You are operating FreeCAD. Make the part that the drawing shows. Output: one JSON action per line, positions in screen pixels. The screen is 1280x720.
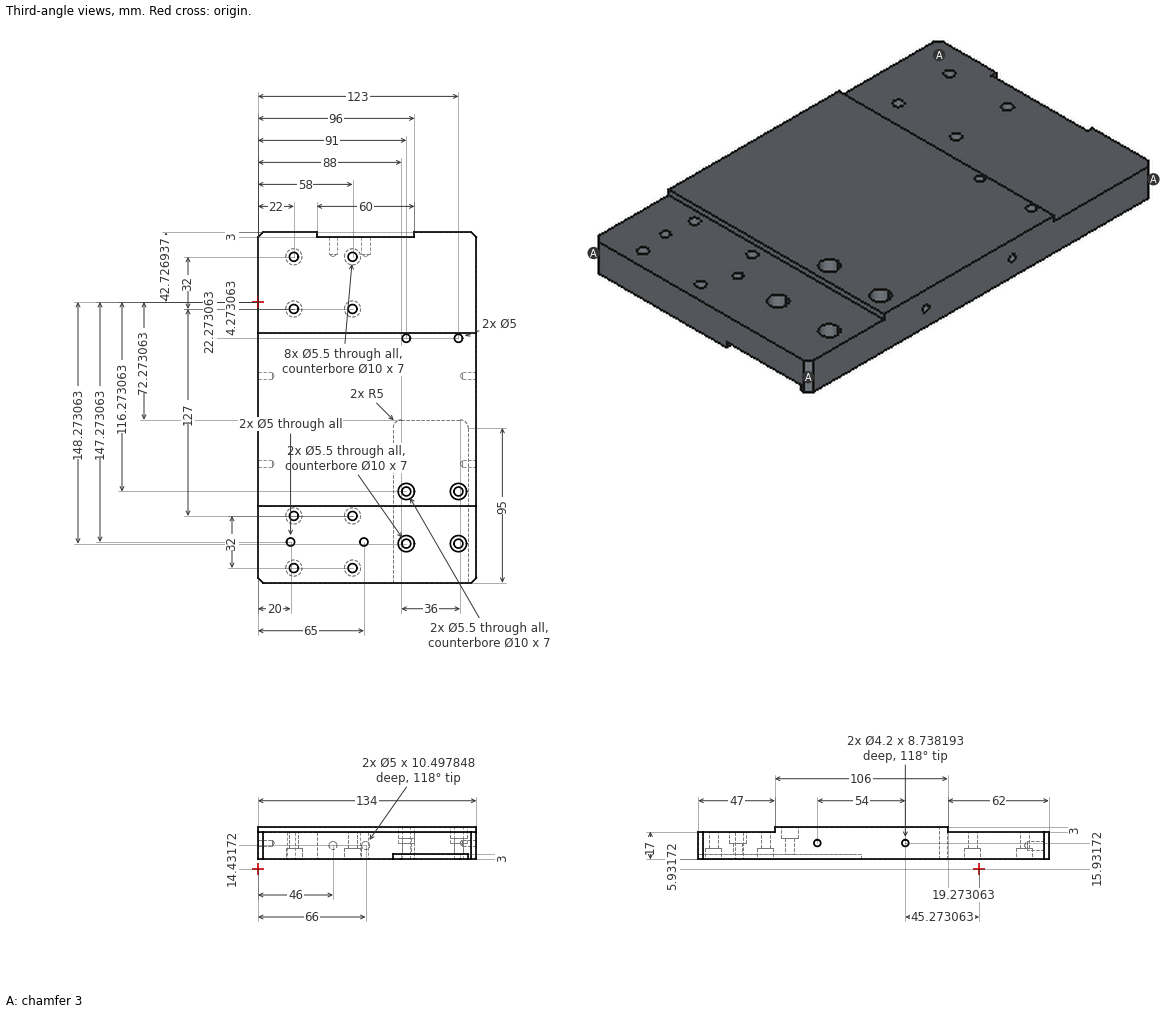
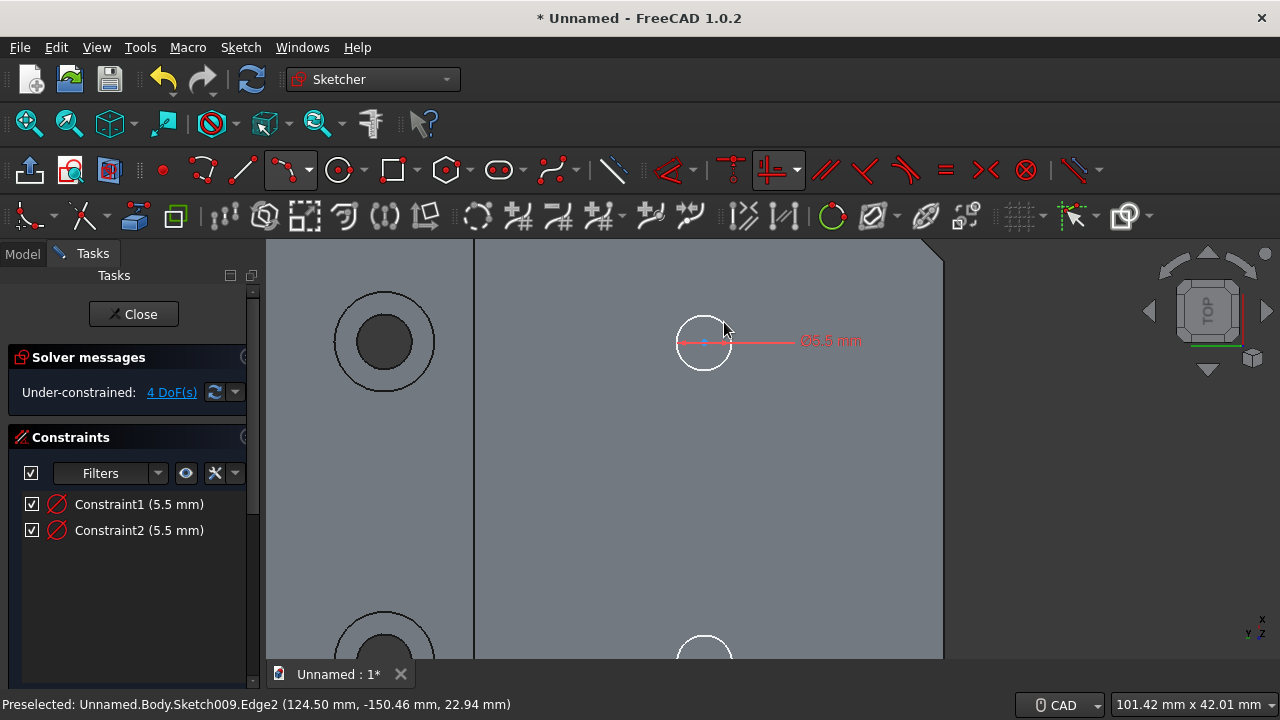
{"action": "scroll", "coordinate": [705, 342], "scroll_direction": "down", "scroll_amount": 2}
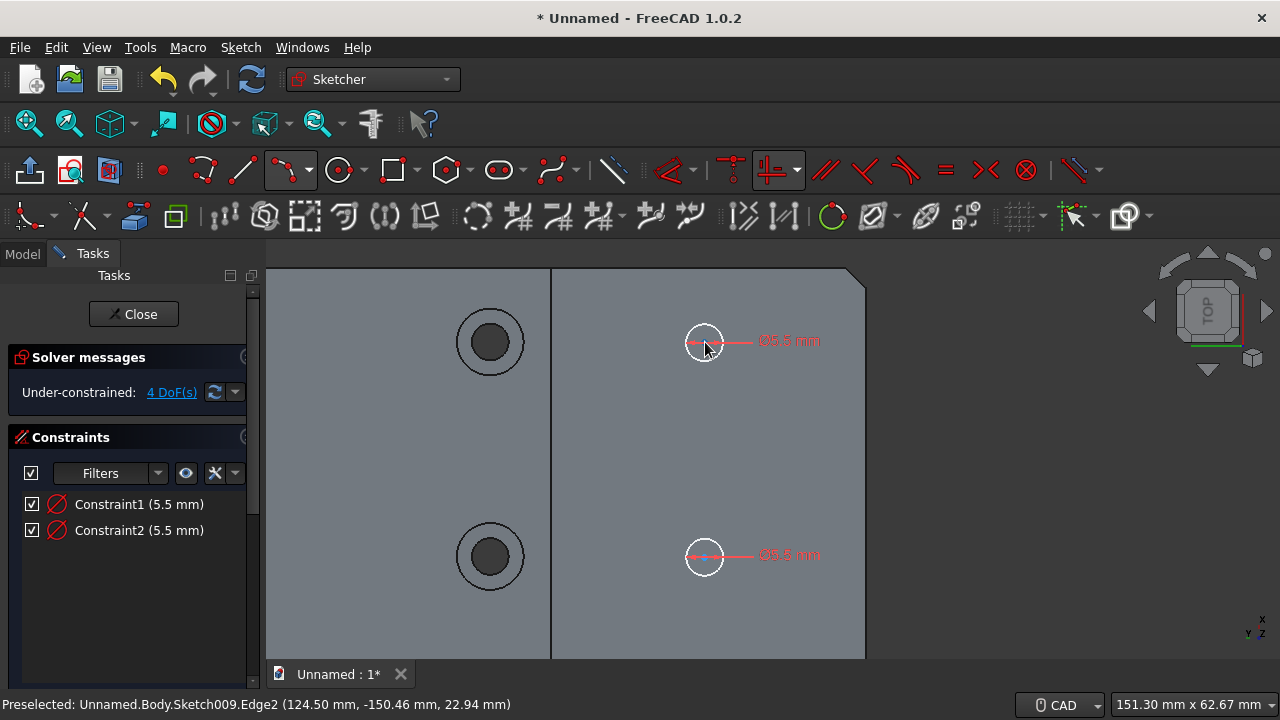
{"action": "left_click", "coordinate": [705, 557]}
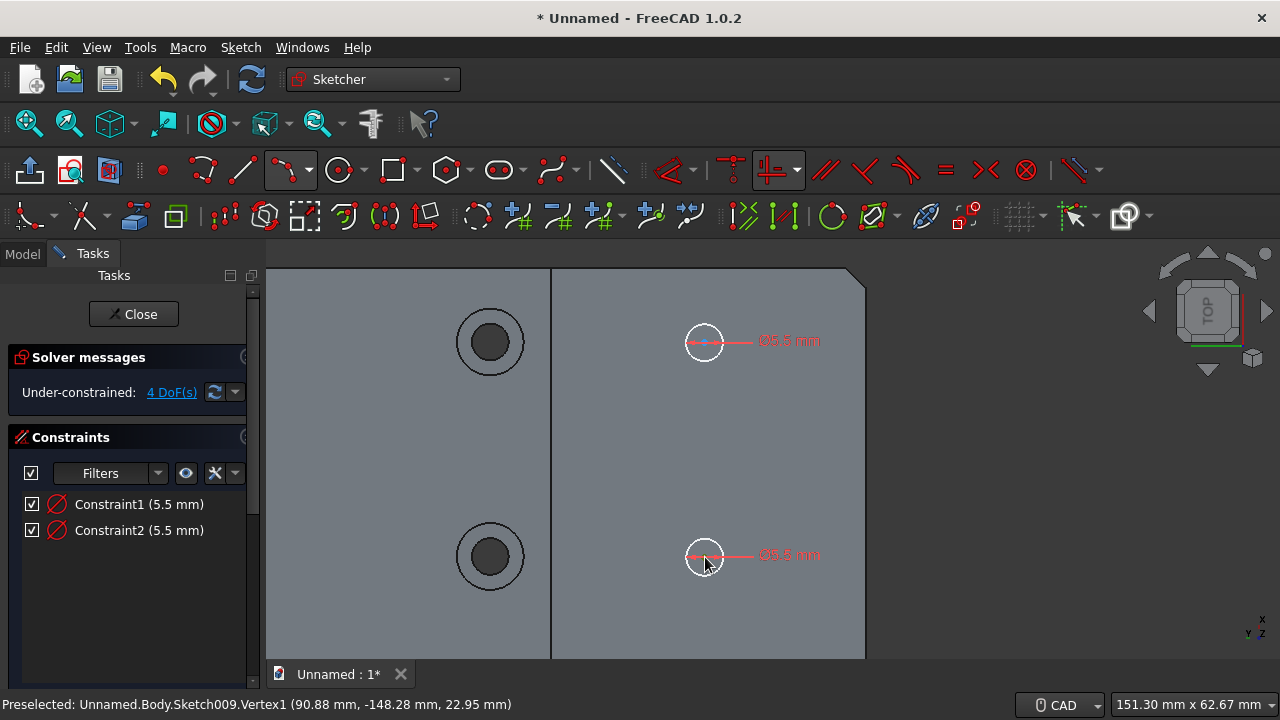
{"action": "left_click", "coordinate": [704, 343]}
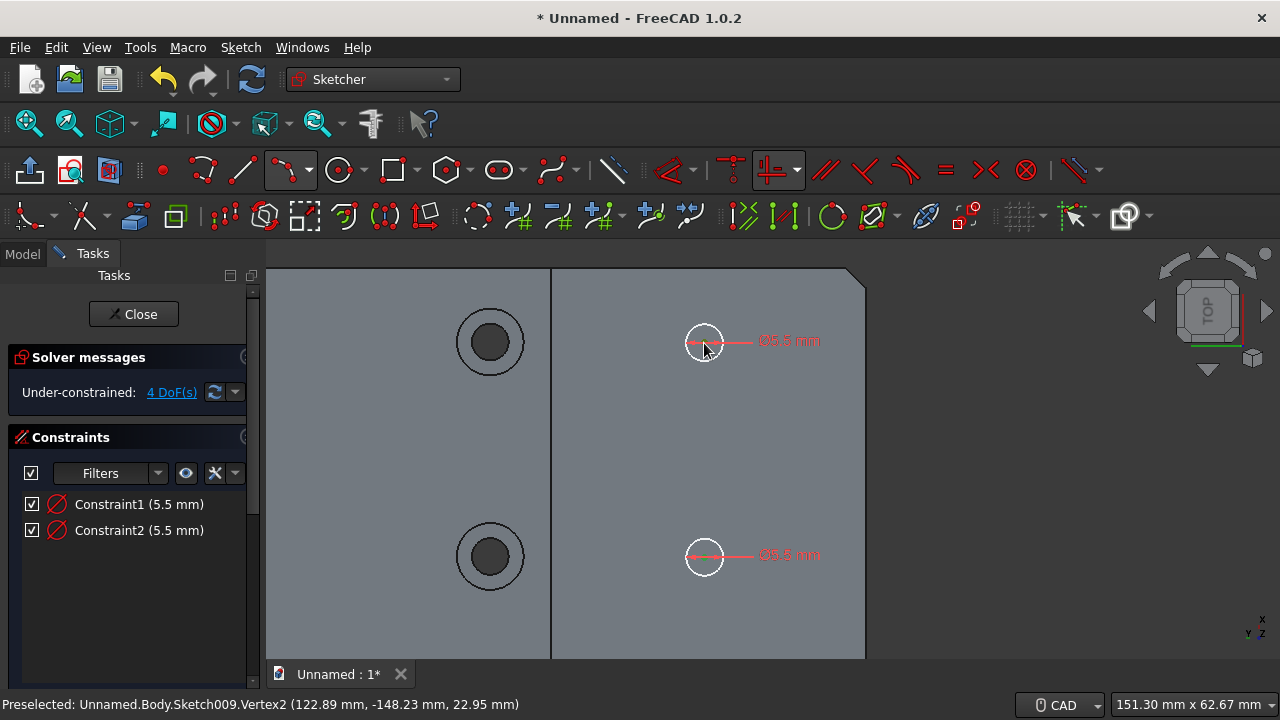
{"action": "key", "text": "v"}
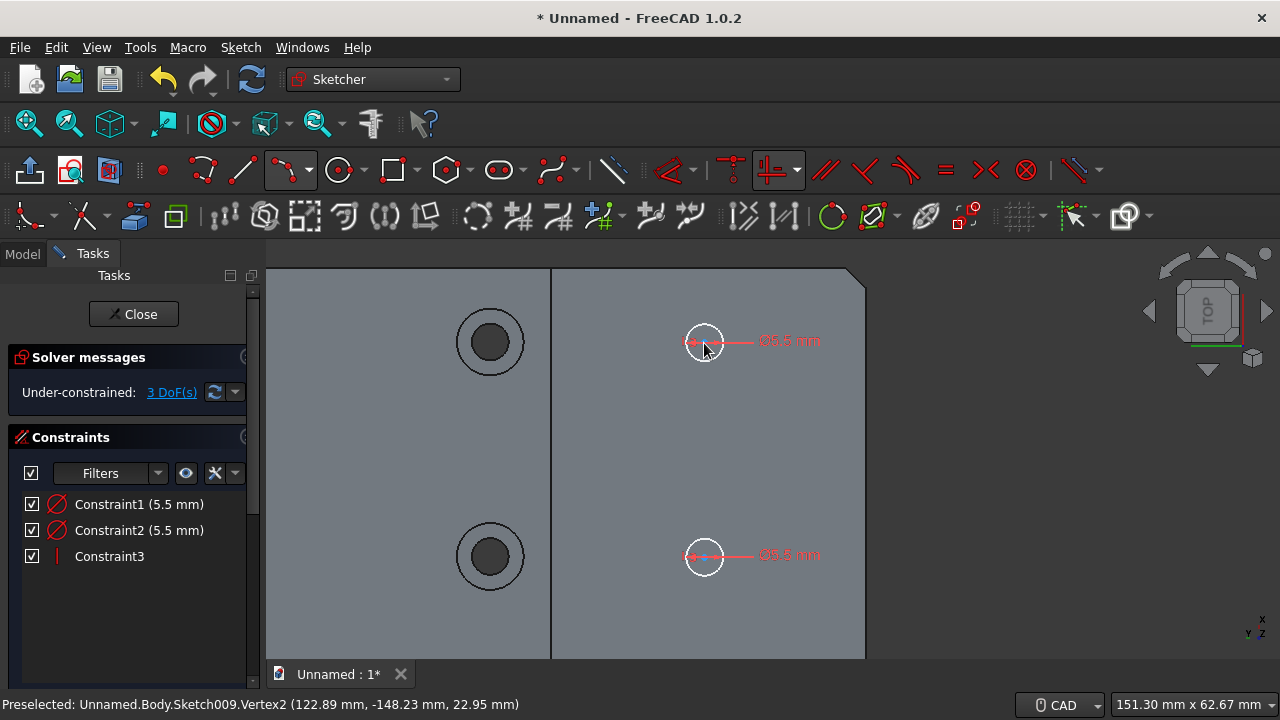
{"action": "left_click", "coordinate": [668, 170]}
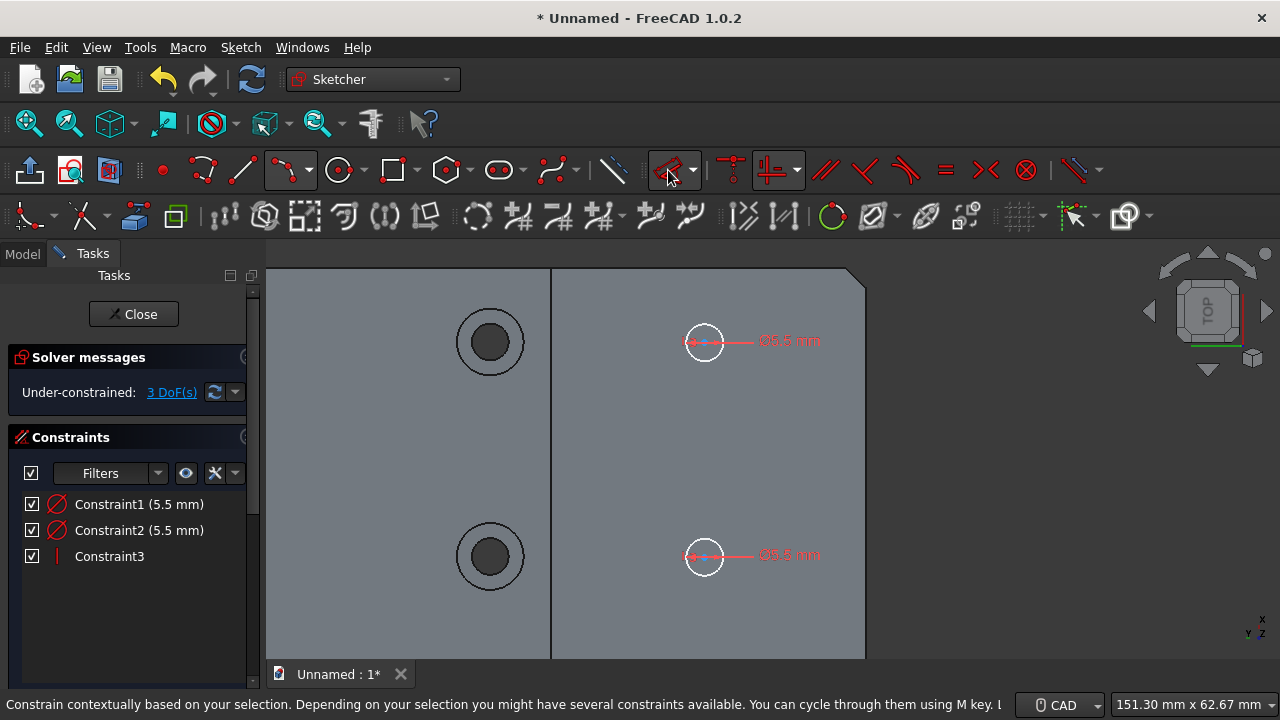
{"action": "left_click", "coordinate": [705, 557]}
{"action": "left_click", "coordinate": [739, 594]}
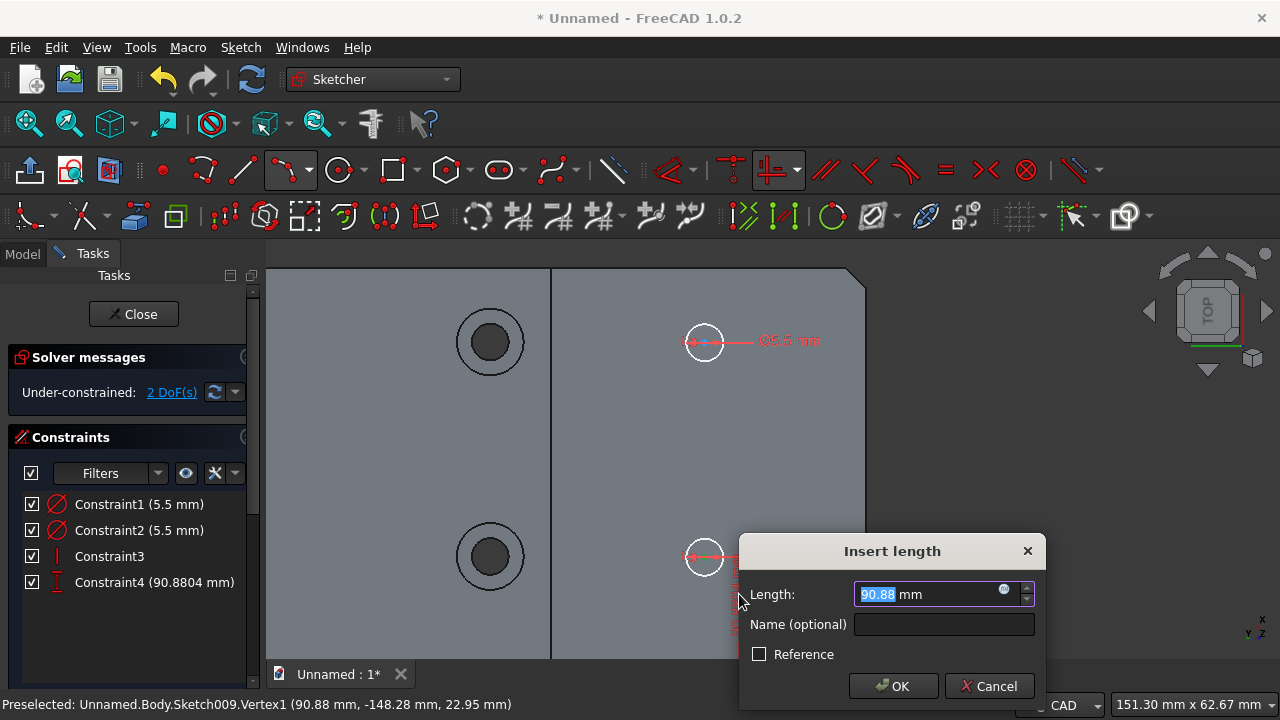
{"action": "type", "text": "91"}
{"action": "key", "text": "Return"}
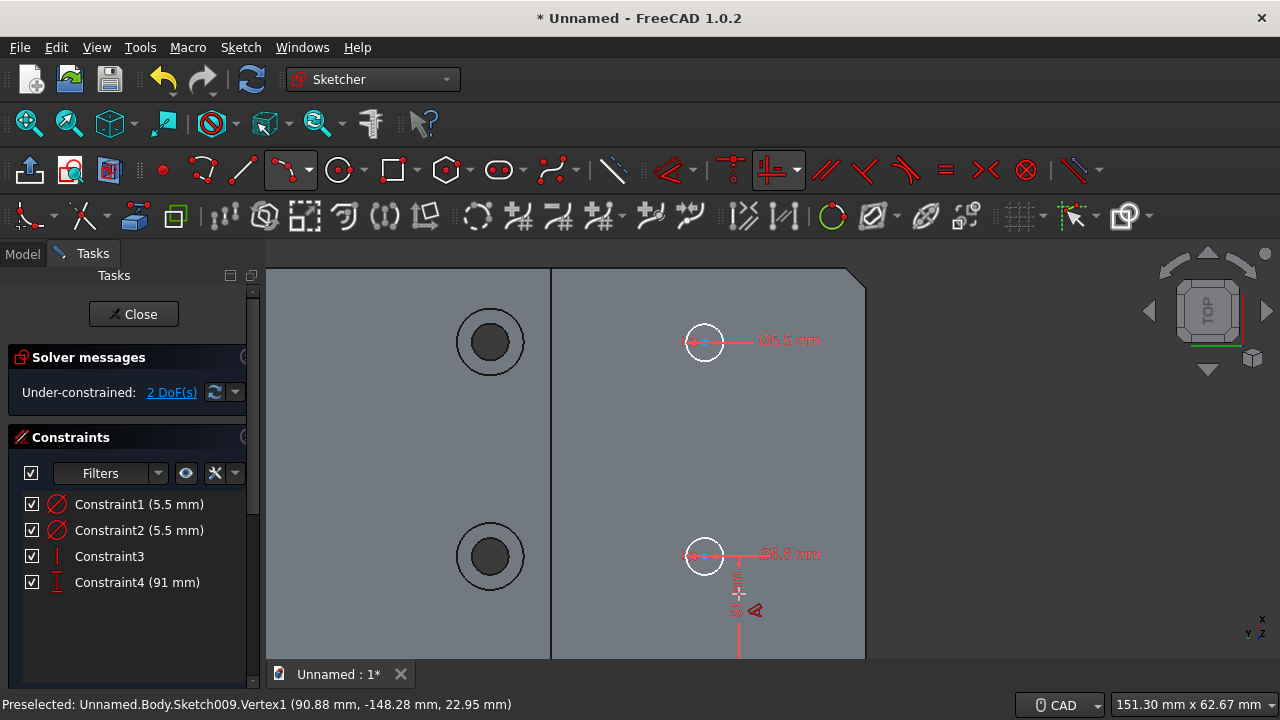
{"action": "left_click", "coordinate": [705, 343]}
{"action": "left_click", "coordinate": [739, 487]}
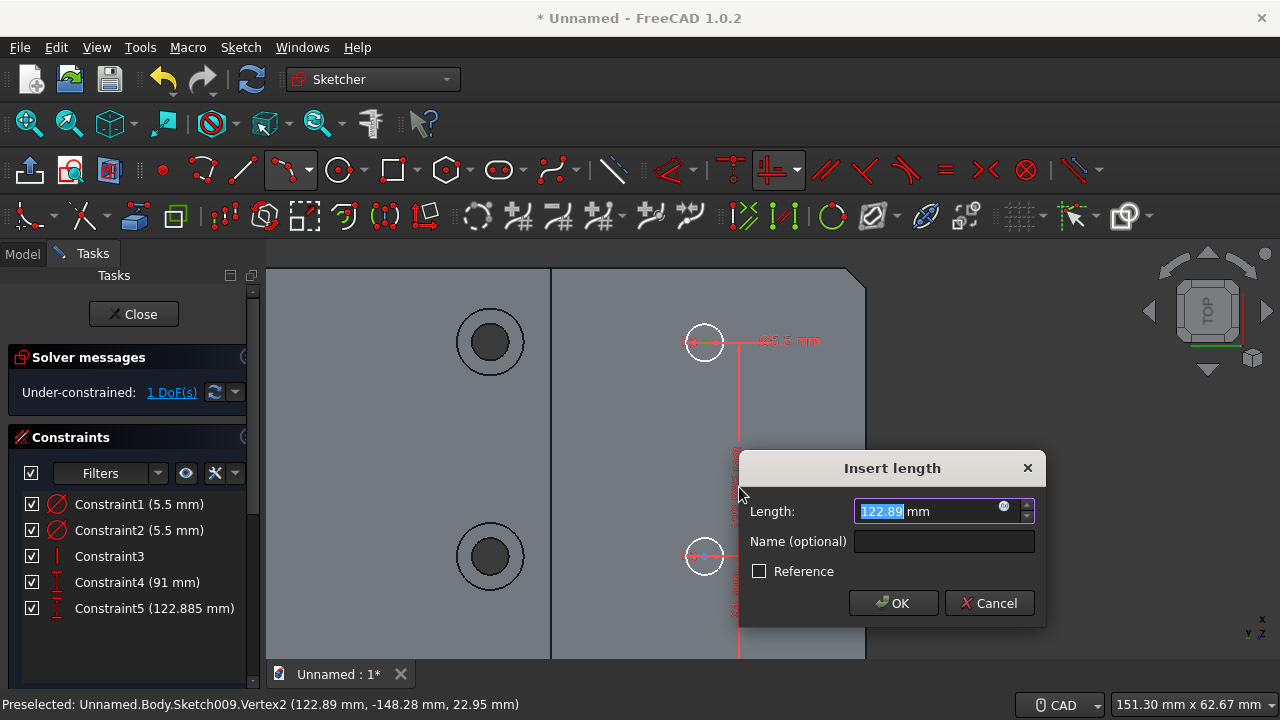
{"action": "type", "text": "123"}
{"action": "key", "text": "Return"}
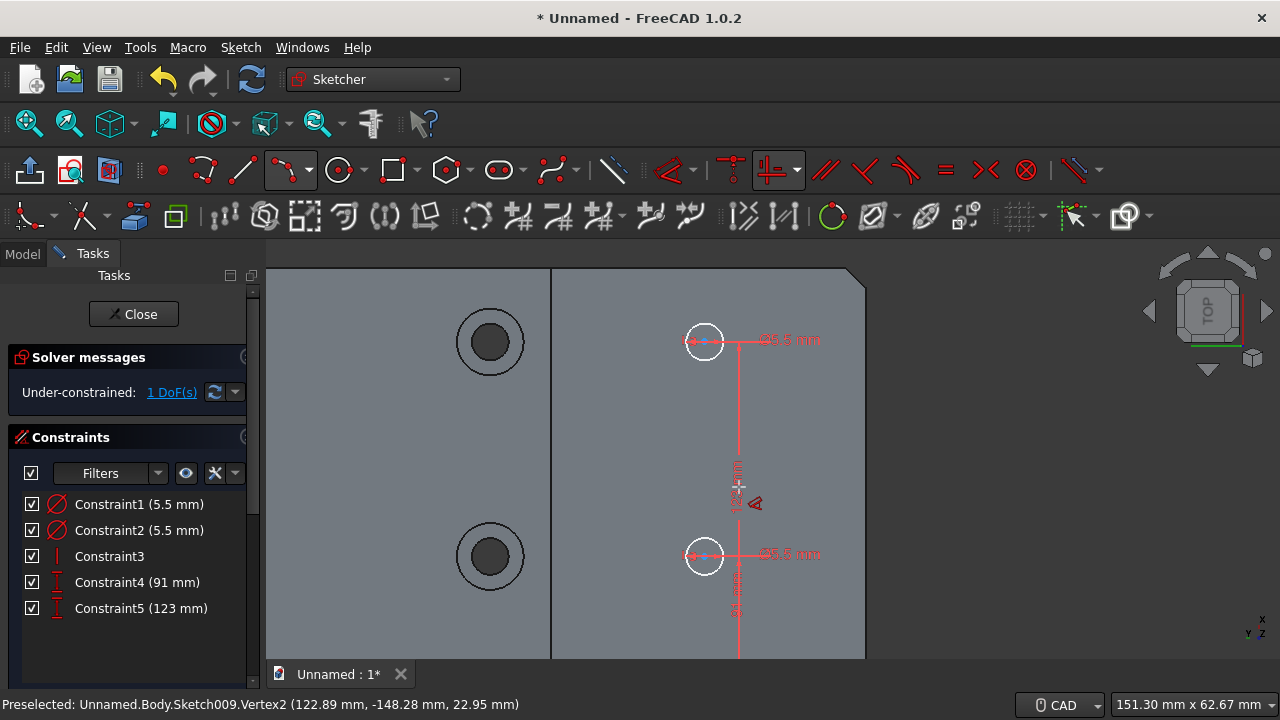
{"action": "left_click", "coordinate": [705, 556]}
{"action": "left_click", "coordinate": [499, 522]}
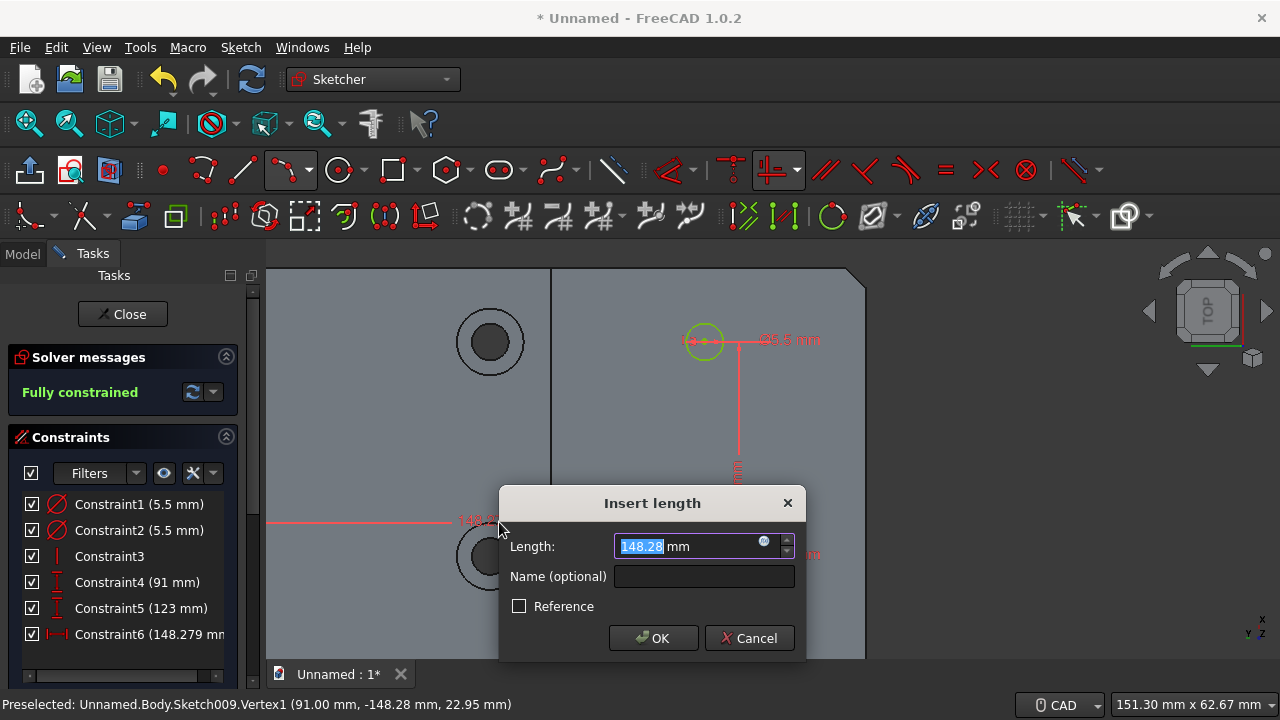
{"action": "type", "text": "148.273063"}
{"action": "key", "text": "Return"}
{"action": "key", "text": "Escape"}